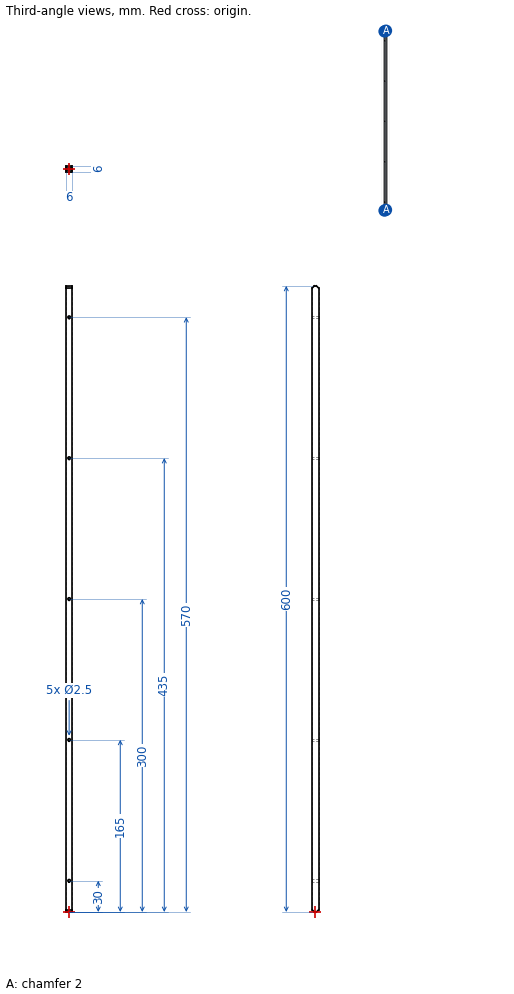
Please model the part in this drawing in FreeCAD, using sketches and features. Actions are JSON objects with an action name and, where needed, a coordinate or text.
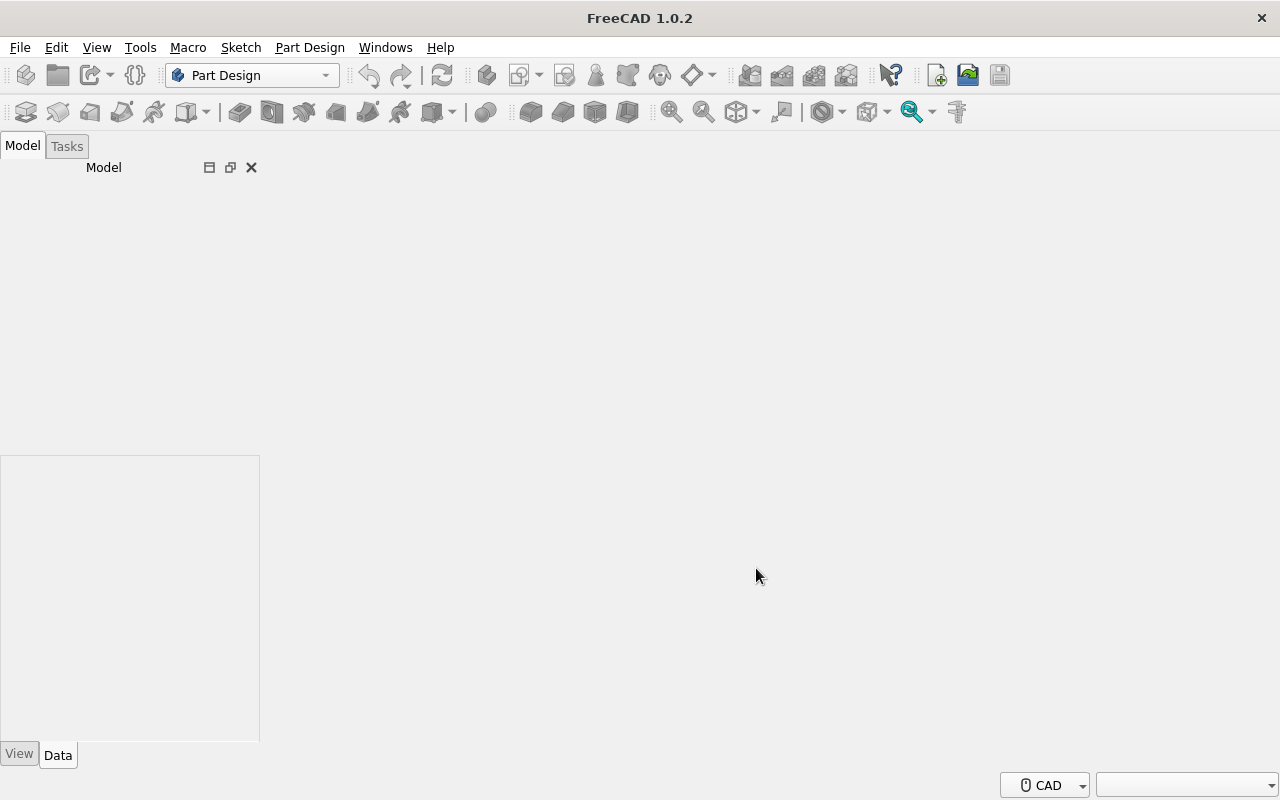
{"action": "left_click", "coordinate": [936, 76]}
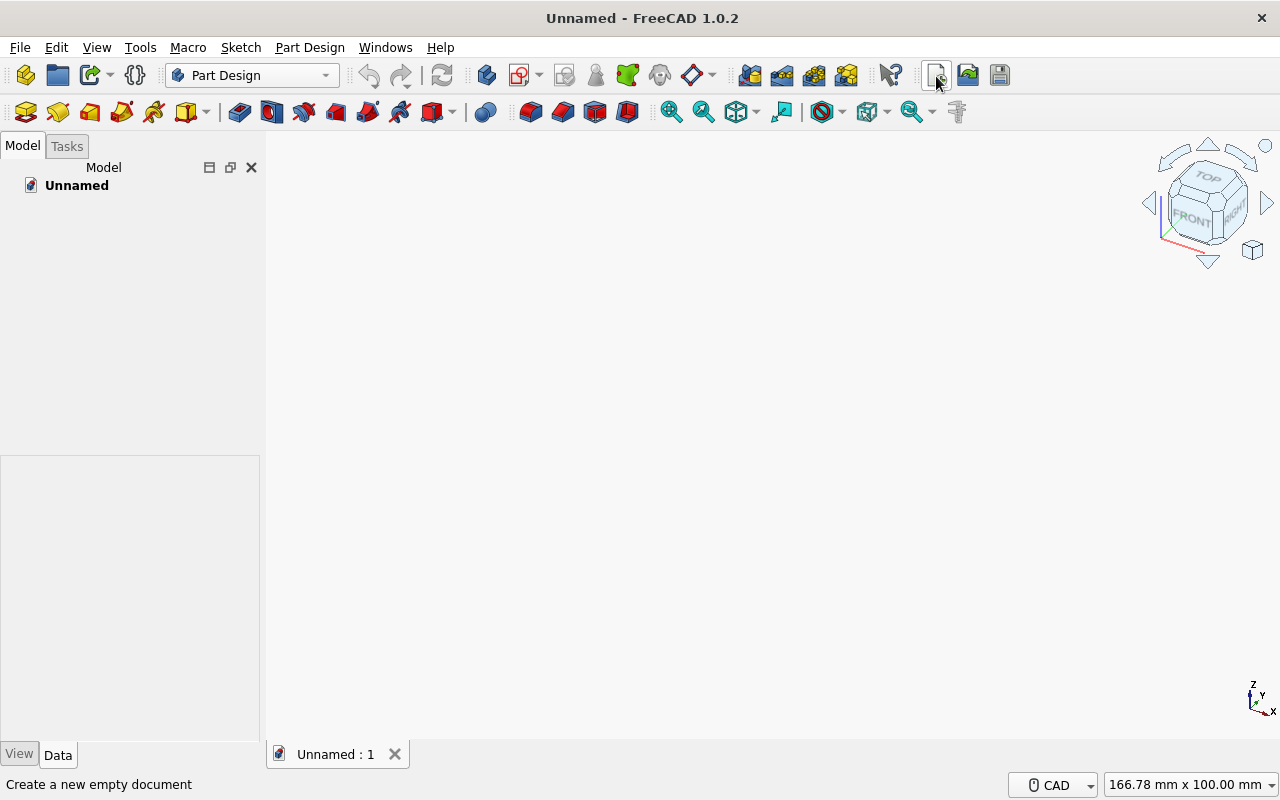
{"action": "left_click", "coordinate": [520, 76]}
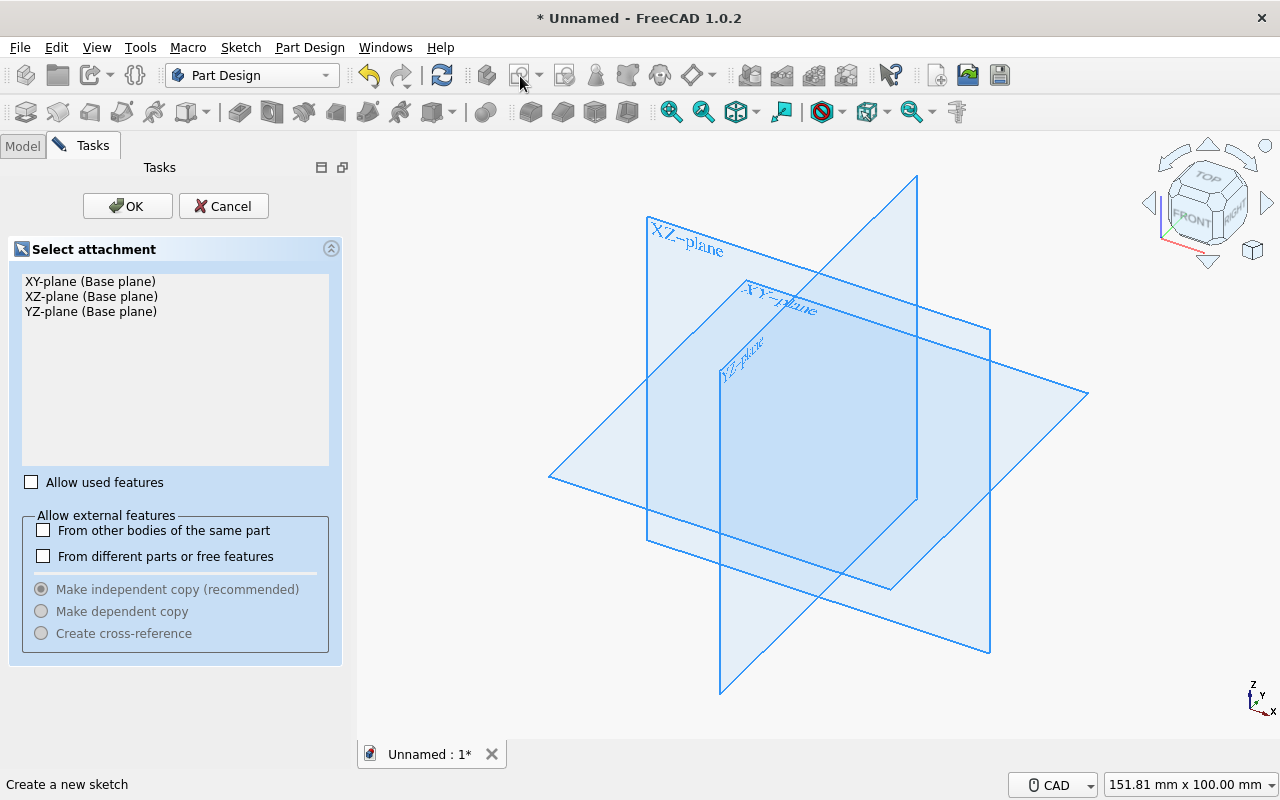
{"action": "left_click", "coordinate": [82, 282]}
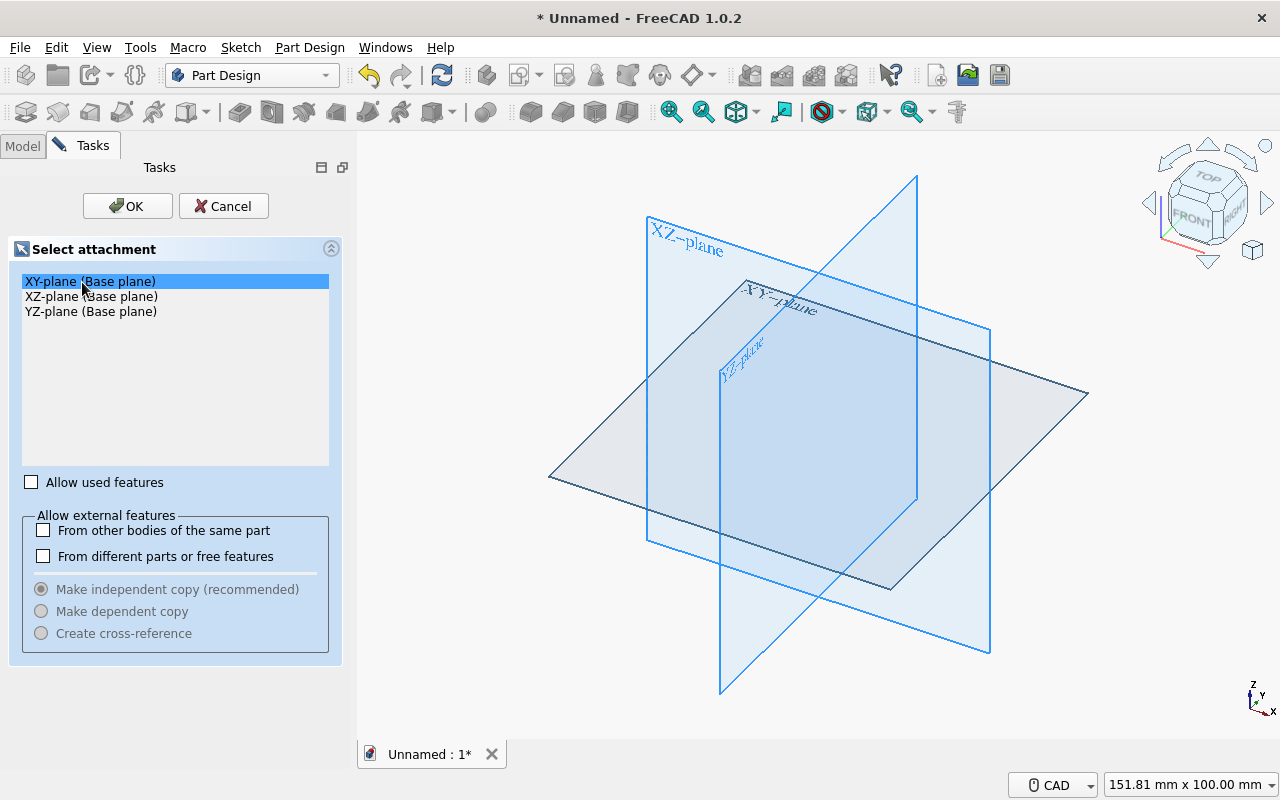
{"action": "left_click", "coordinate": [128, 206]}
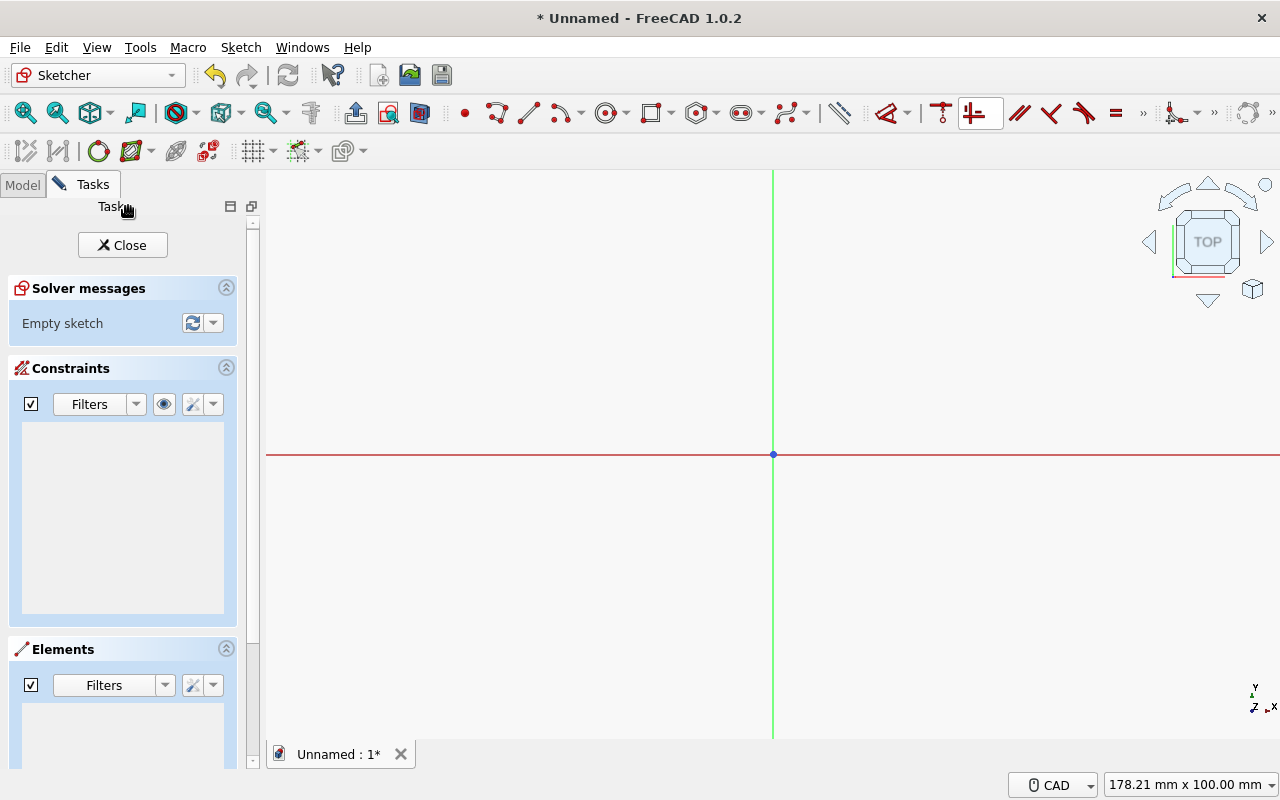
{"action": "scroll", "coordinate": [780, 455], "scroll_direction": "up", "scroll_amount": 12}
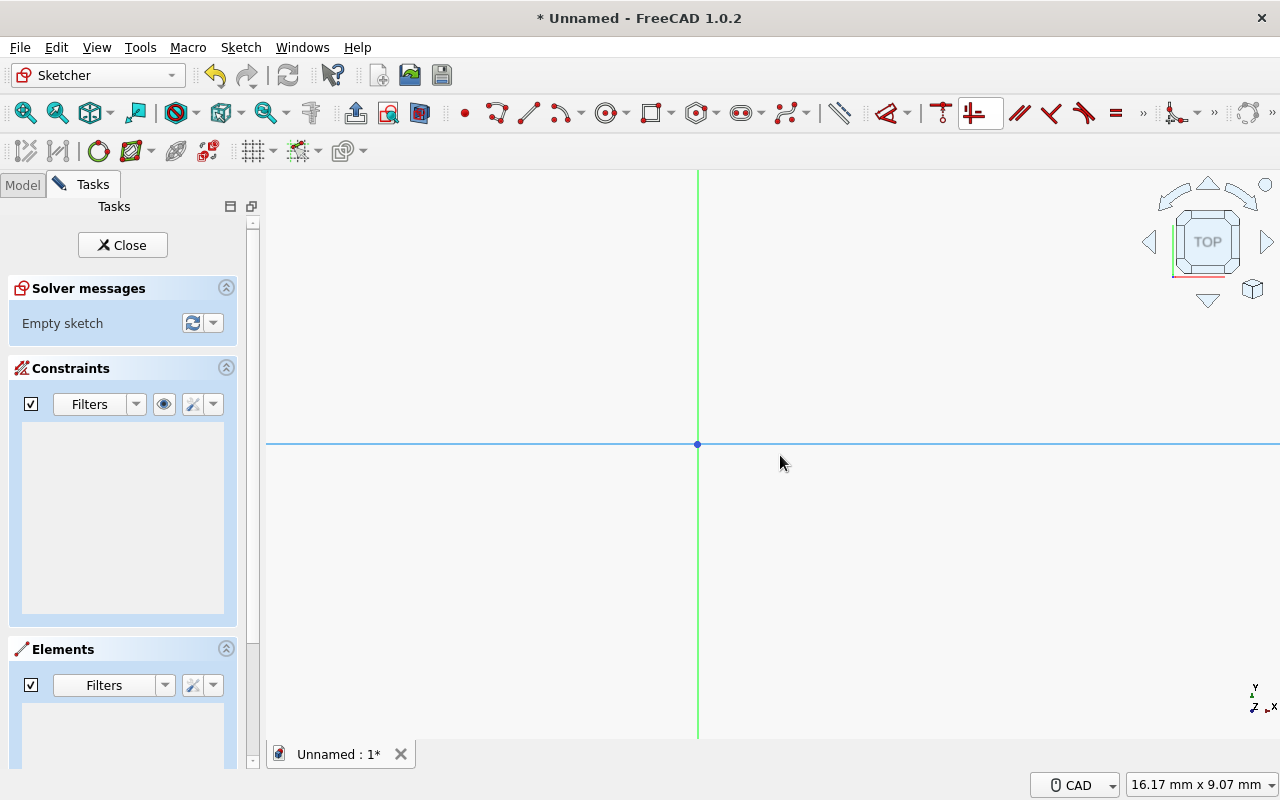
{"action": "key", "text": "g v"}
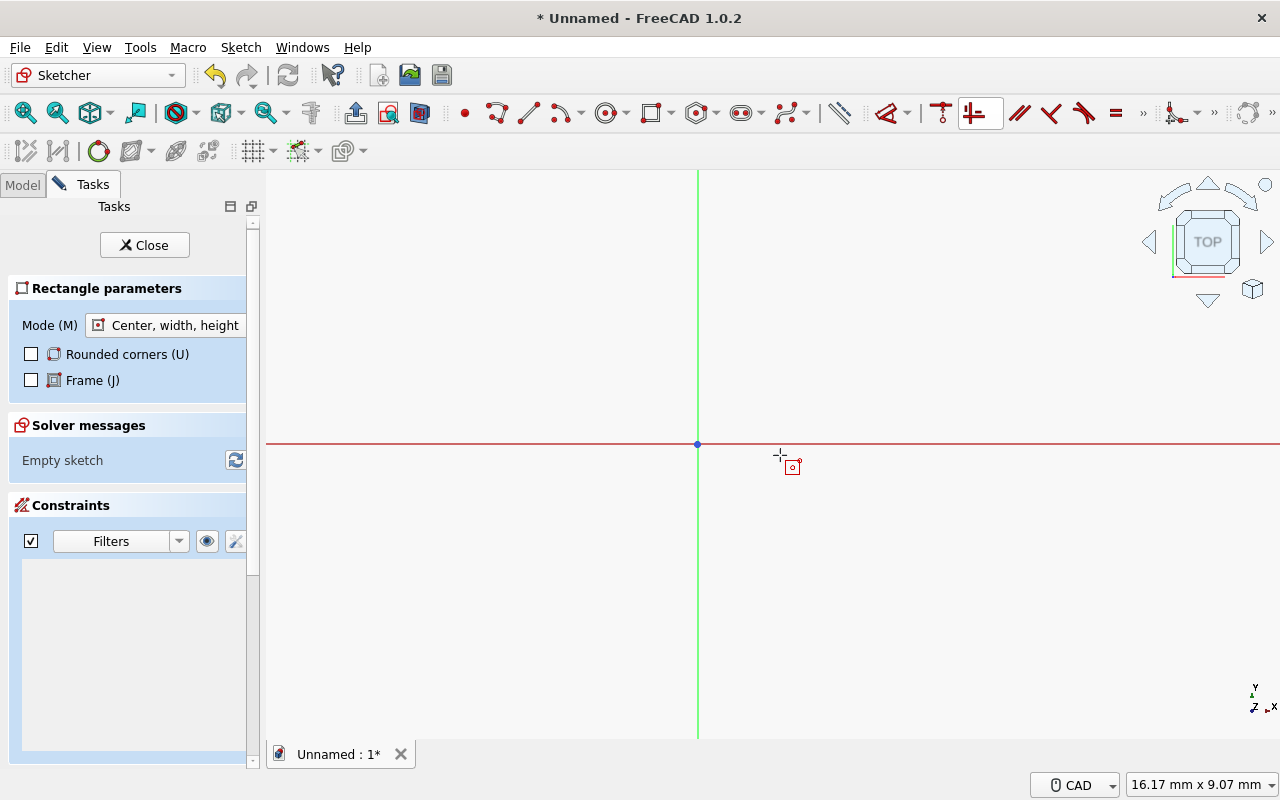
{"action": "left_click", "coordinate": [698, 444]}
{"action": "mouse_move", "coordinate": [886, 256]}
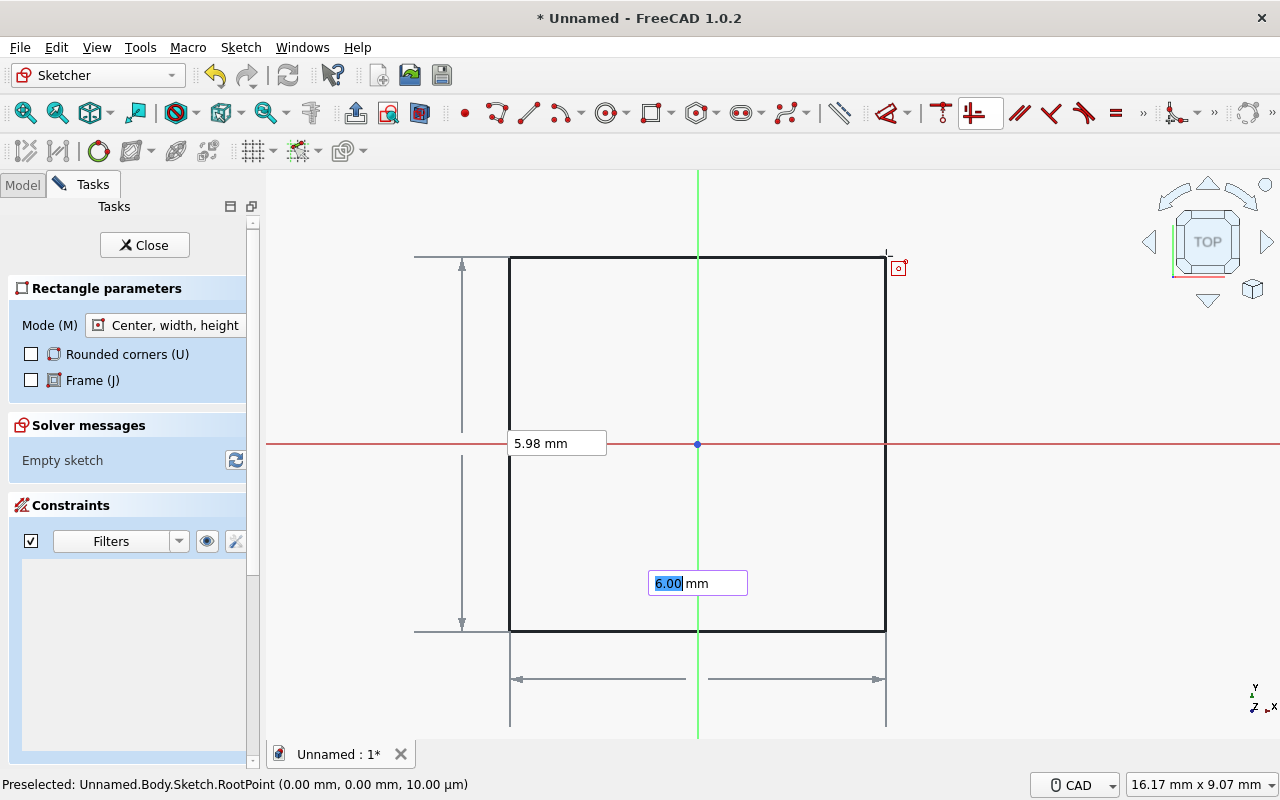
{"action": "type", "text": "6"}
{"action": "key", "text": "Tab"}
{"action": "type", "text": "6"}
{"action": "key", "text": "Return"}
{"action": "key", "text": "Escape"}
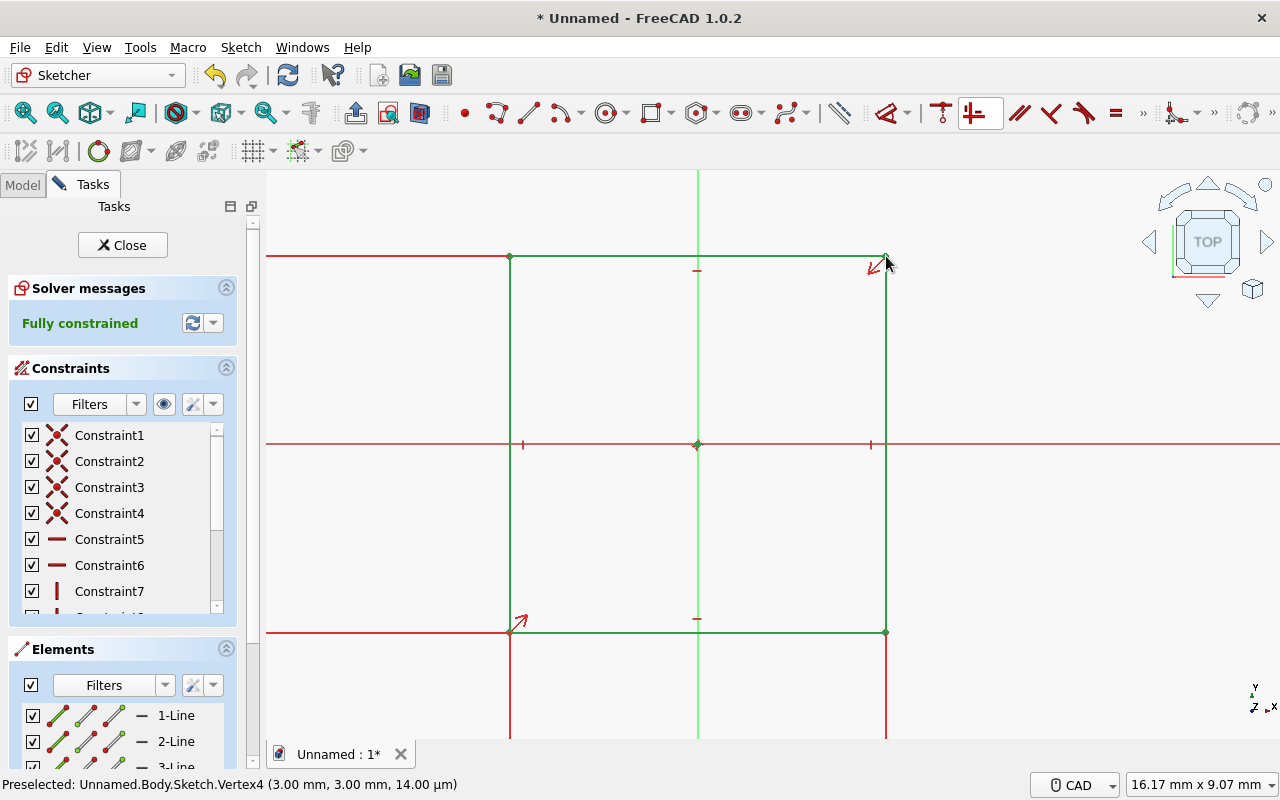
{"action": "left_click", "coordinate": [123, 245]}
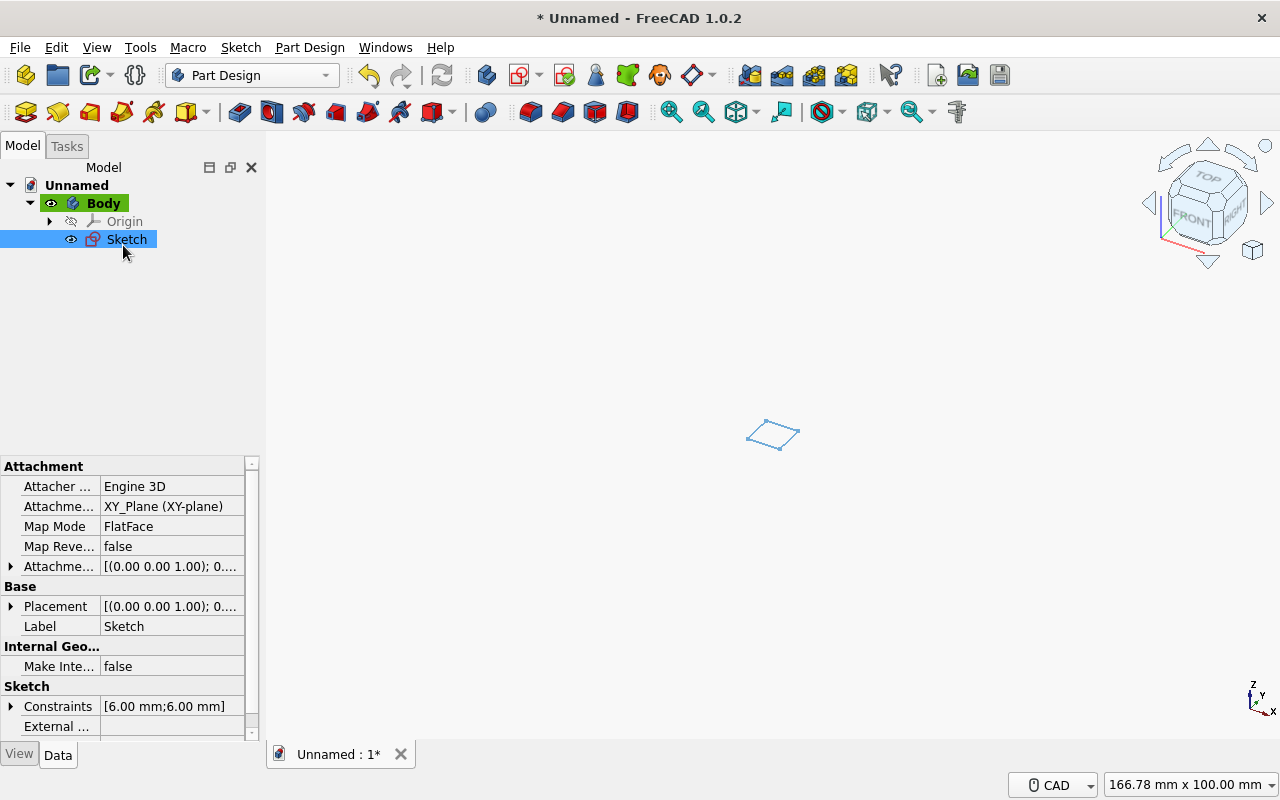
{"action": "left_click", "coordinate": [26, 112]}